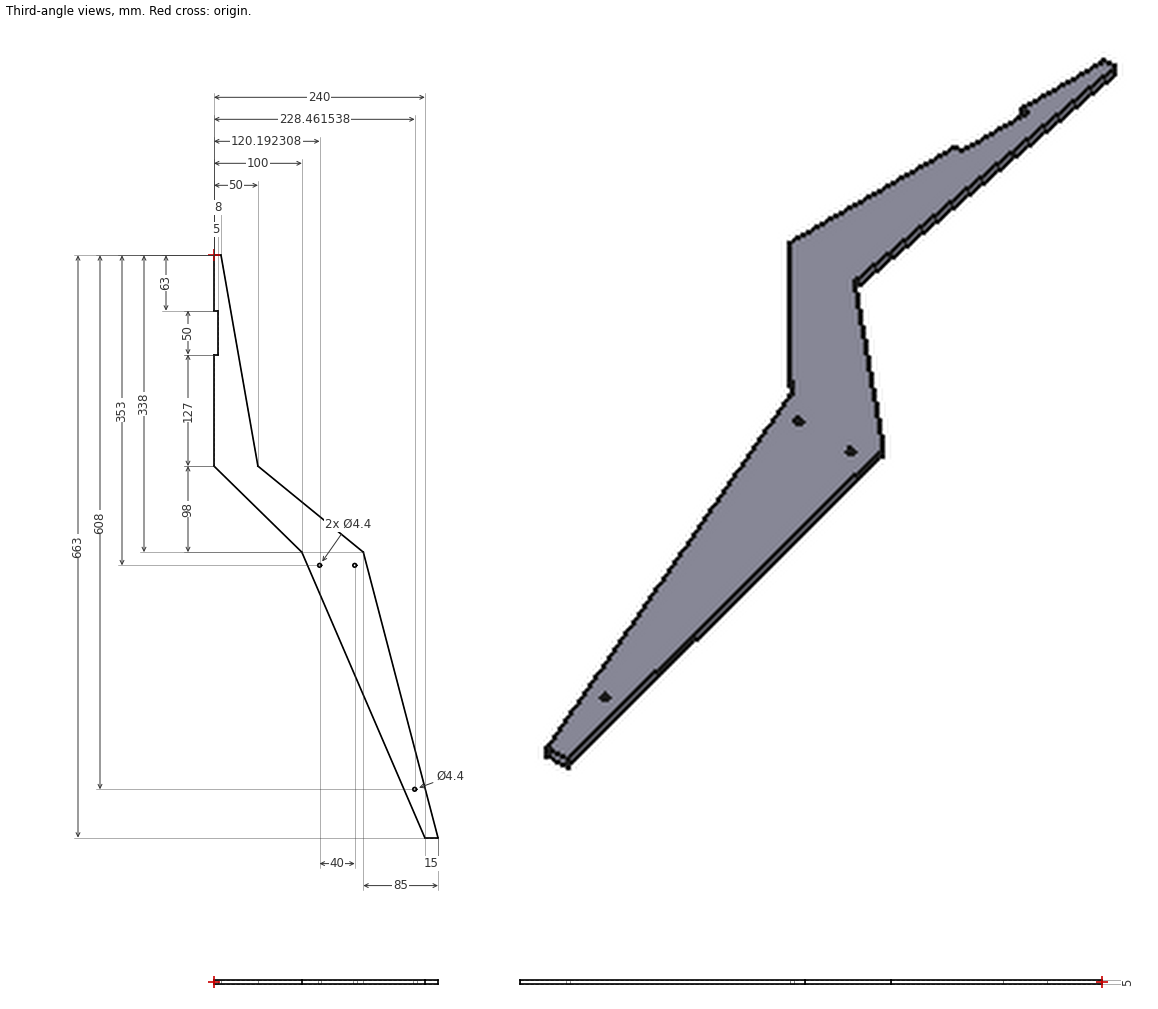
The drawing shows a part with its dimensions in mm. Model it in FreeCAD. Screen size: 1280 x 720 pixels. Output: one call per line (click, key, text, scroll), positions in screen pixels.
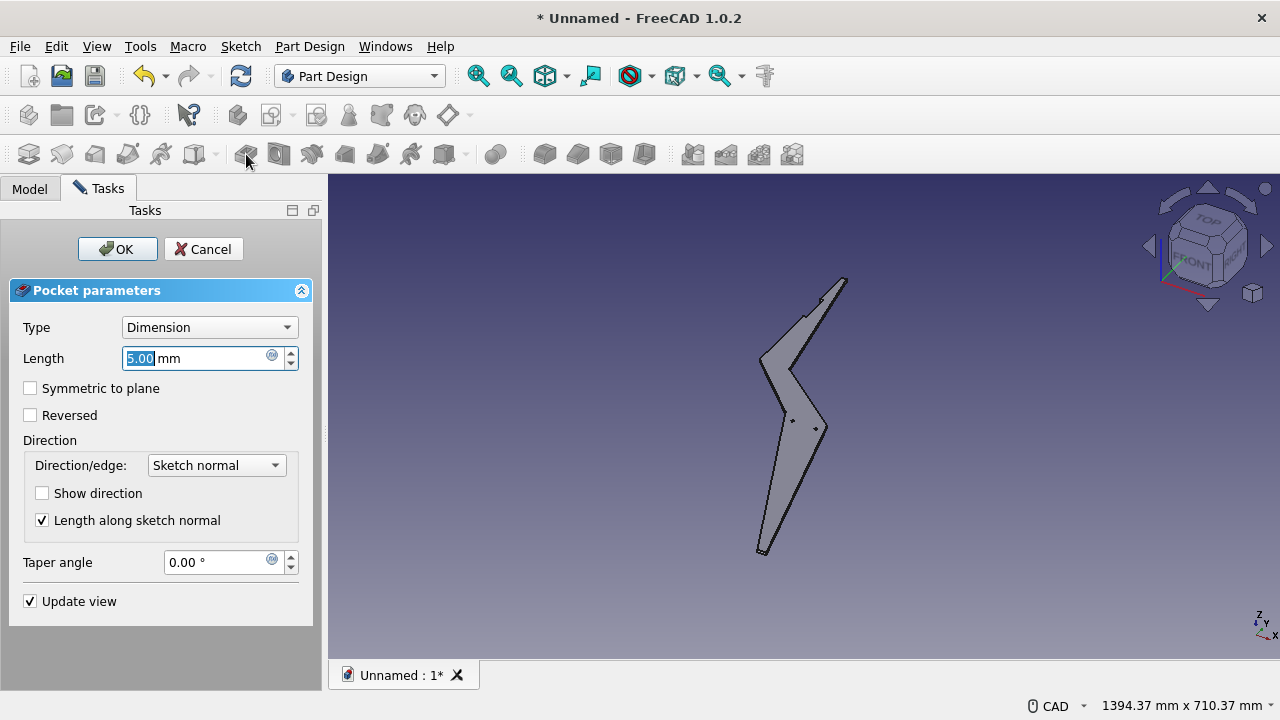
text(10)
key(Tab)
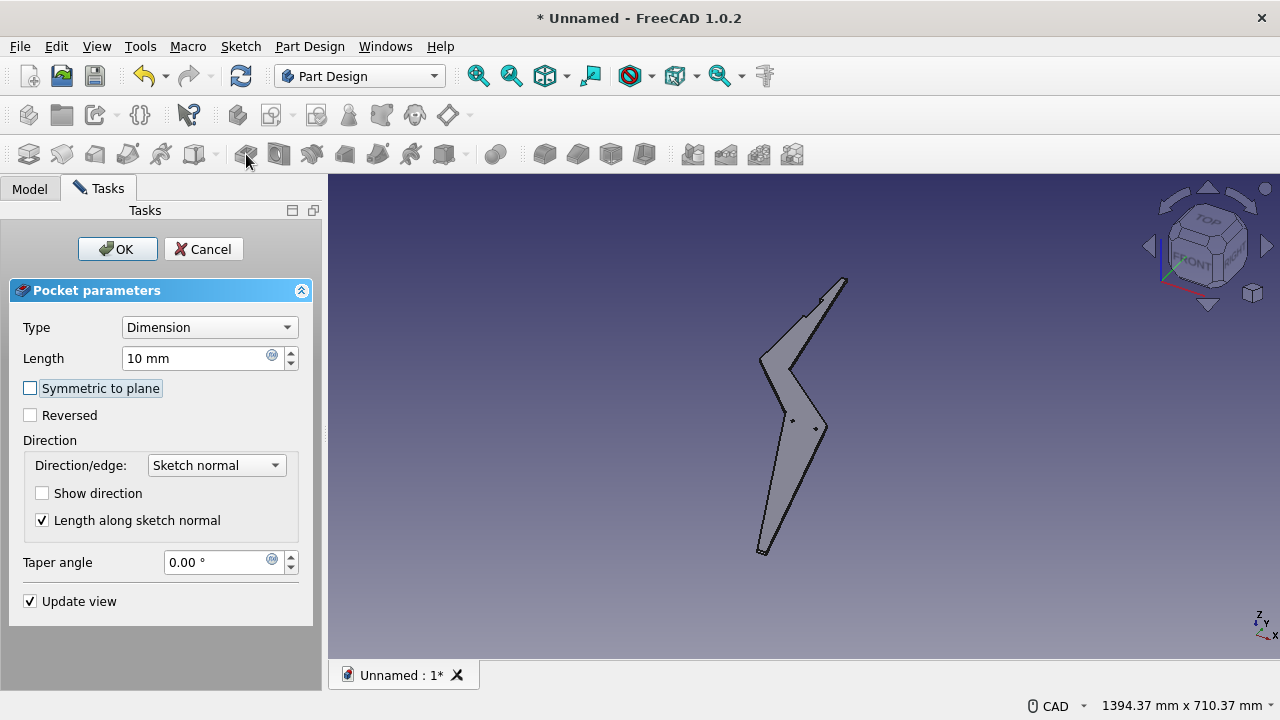
click(118, 249)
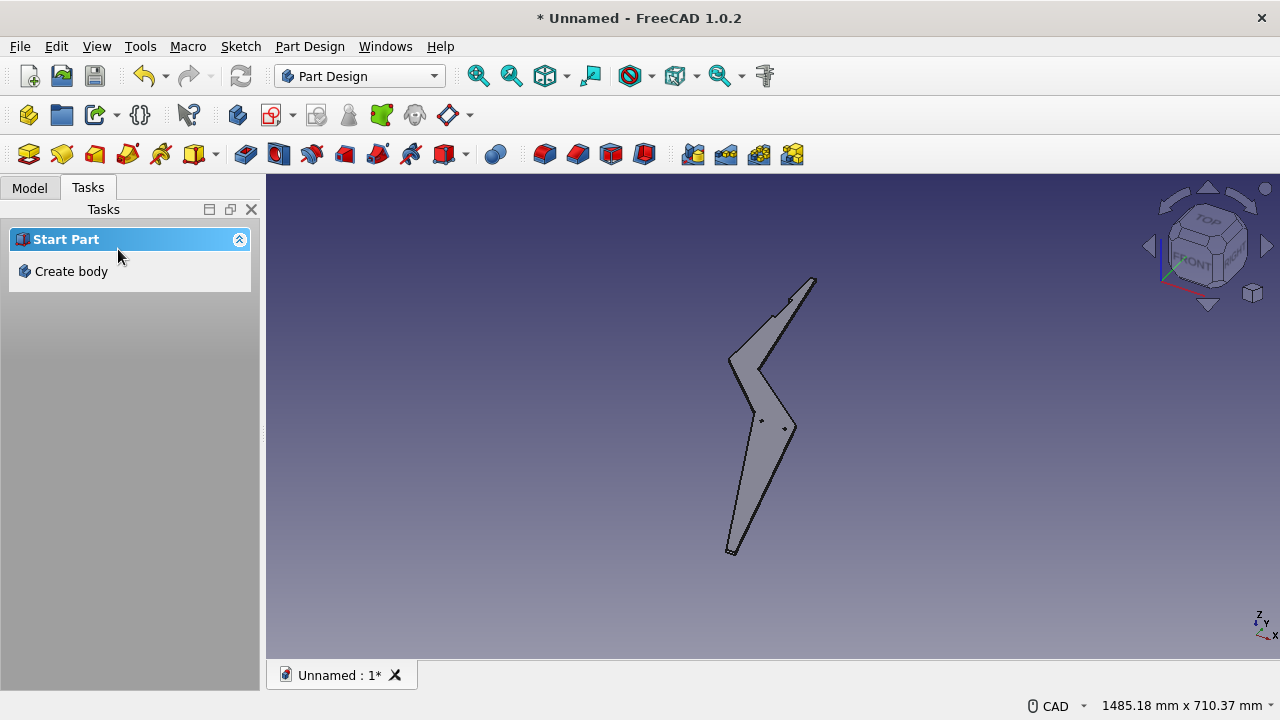
click(762, 453)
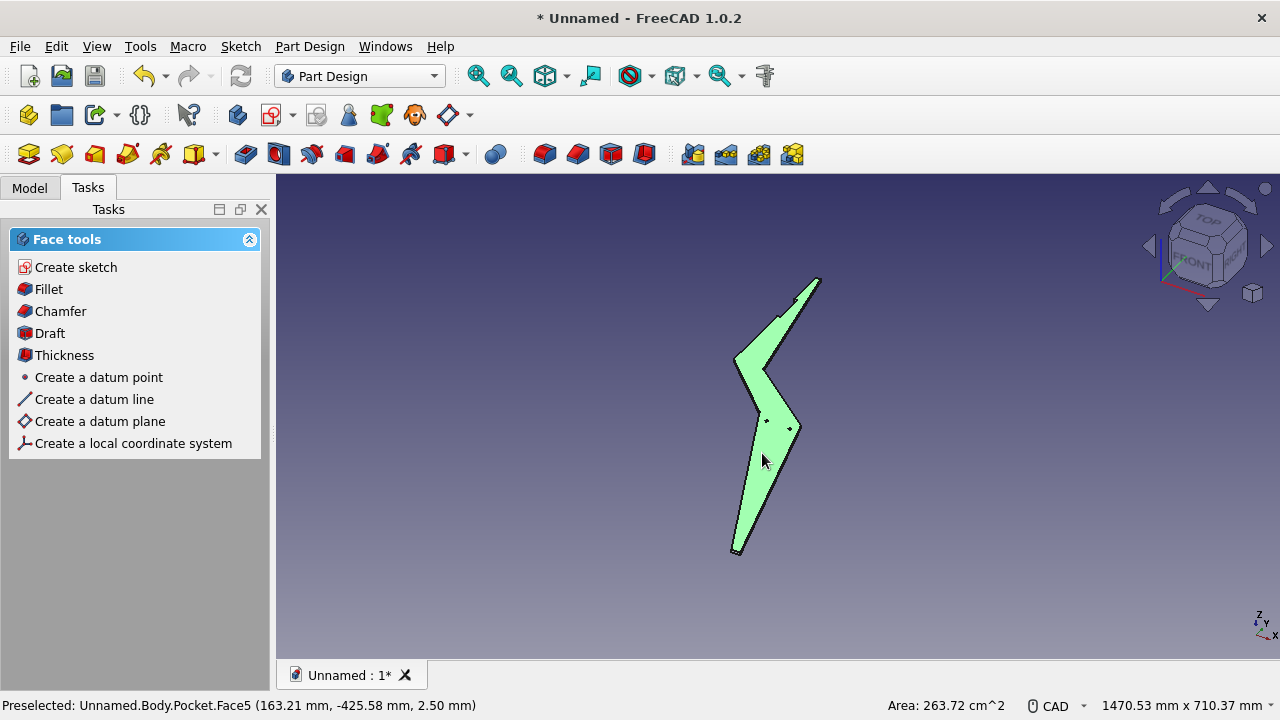
click(270, 116)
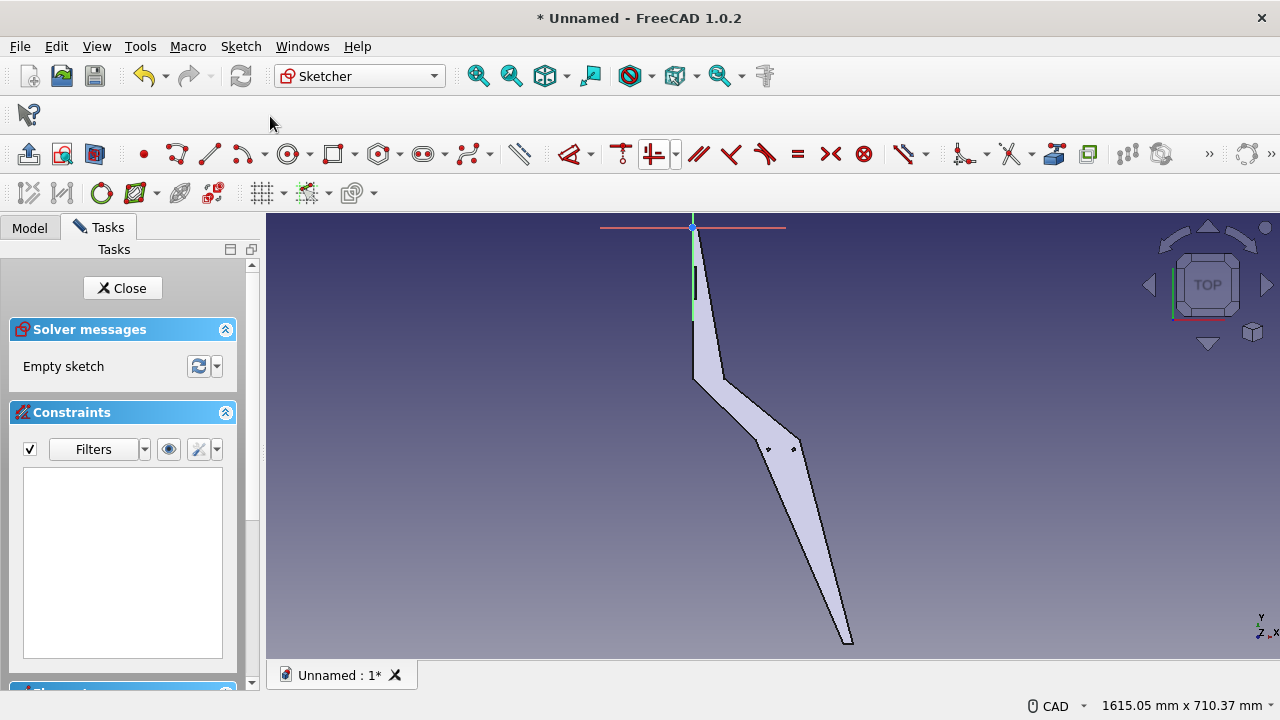
scroll(843, 619, up, 15)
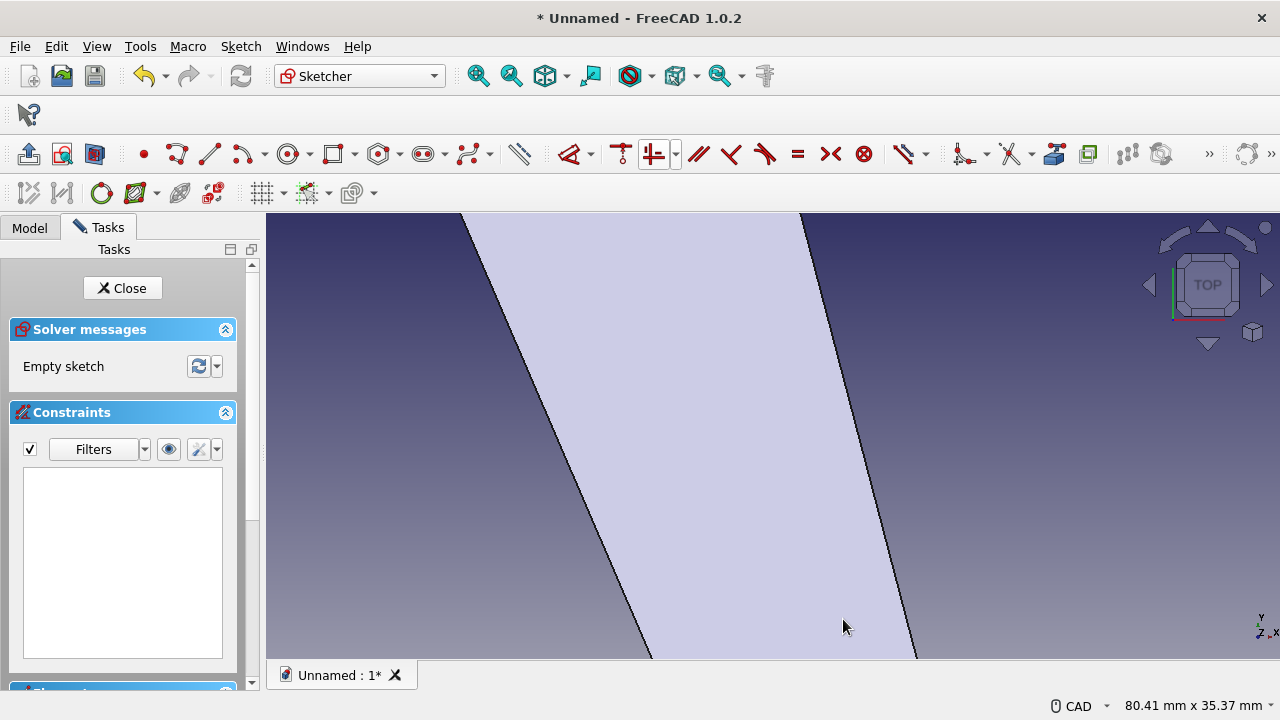
scroll(698, 407, up, 8)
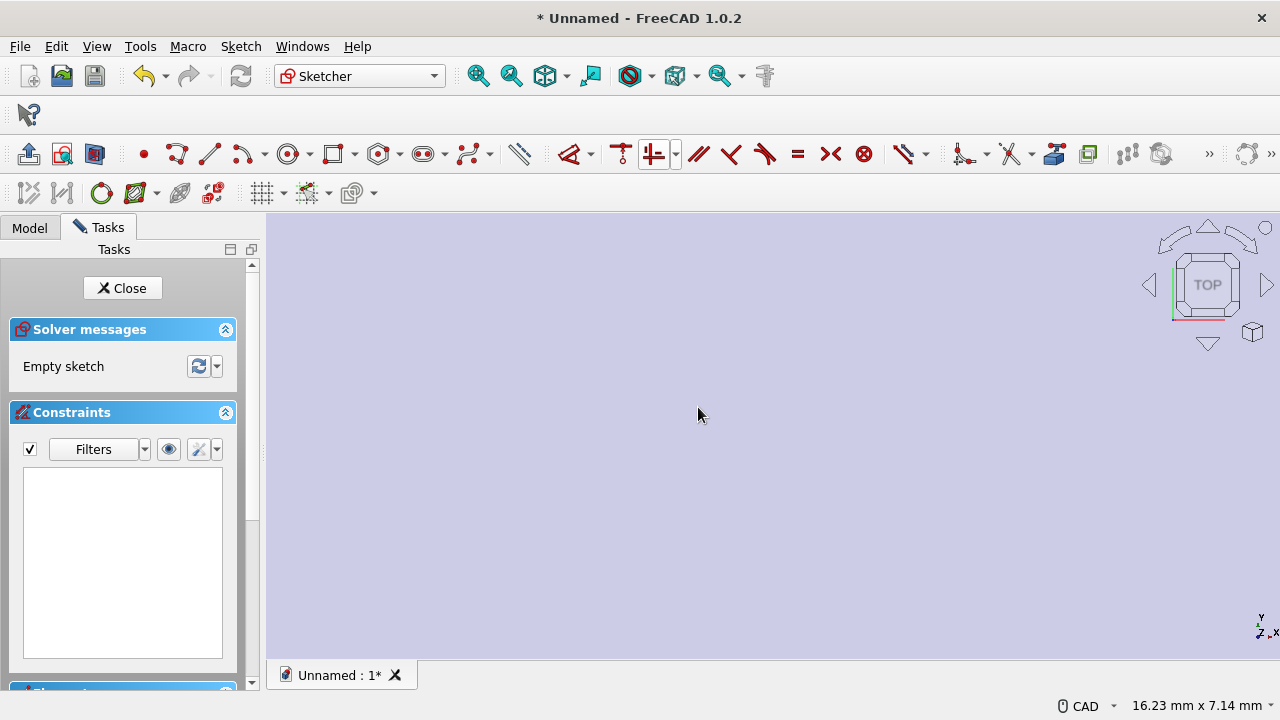
click(288, 154)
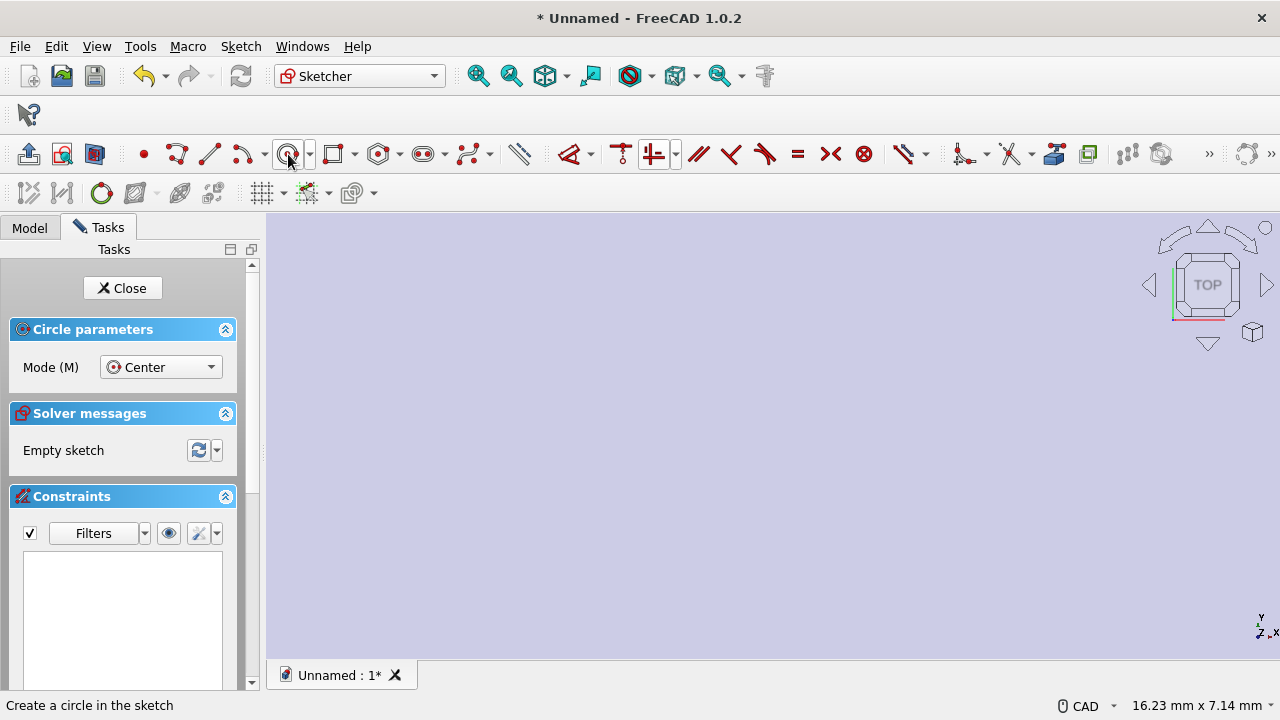
click(703, 434)
click(800, 337)
key(Escape)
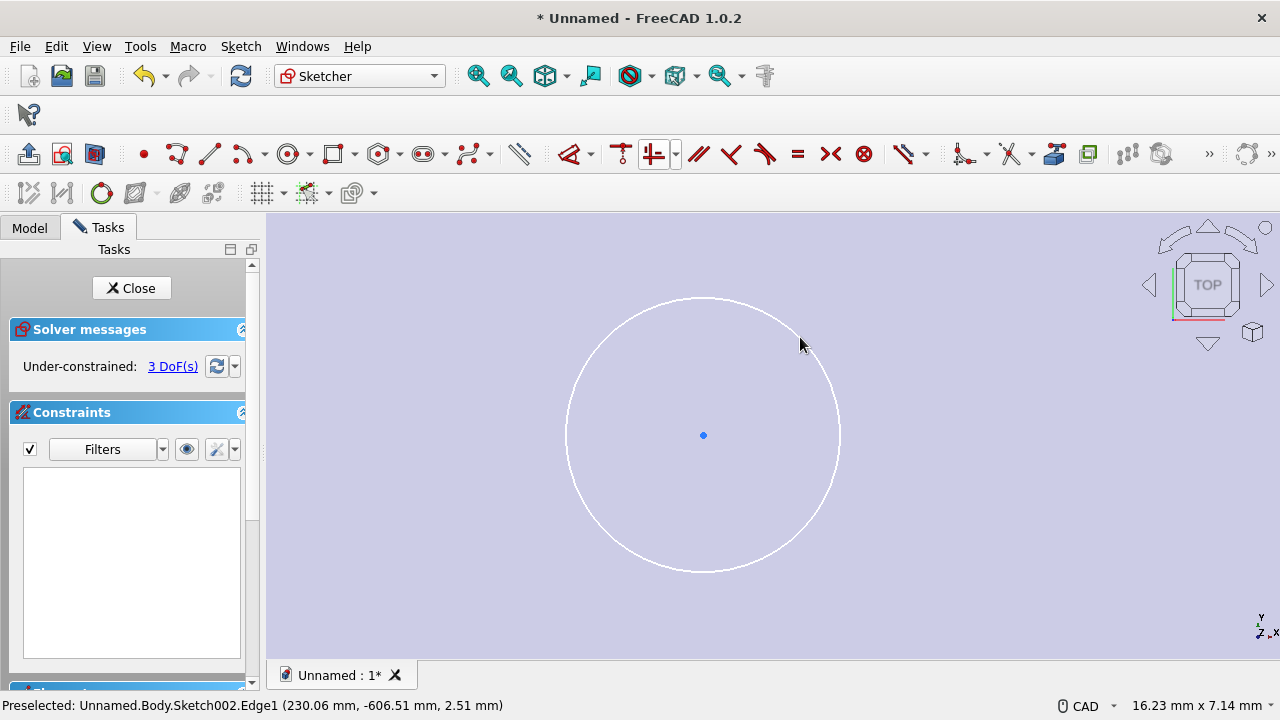
click(568, 154)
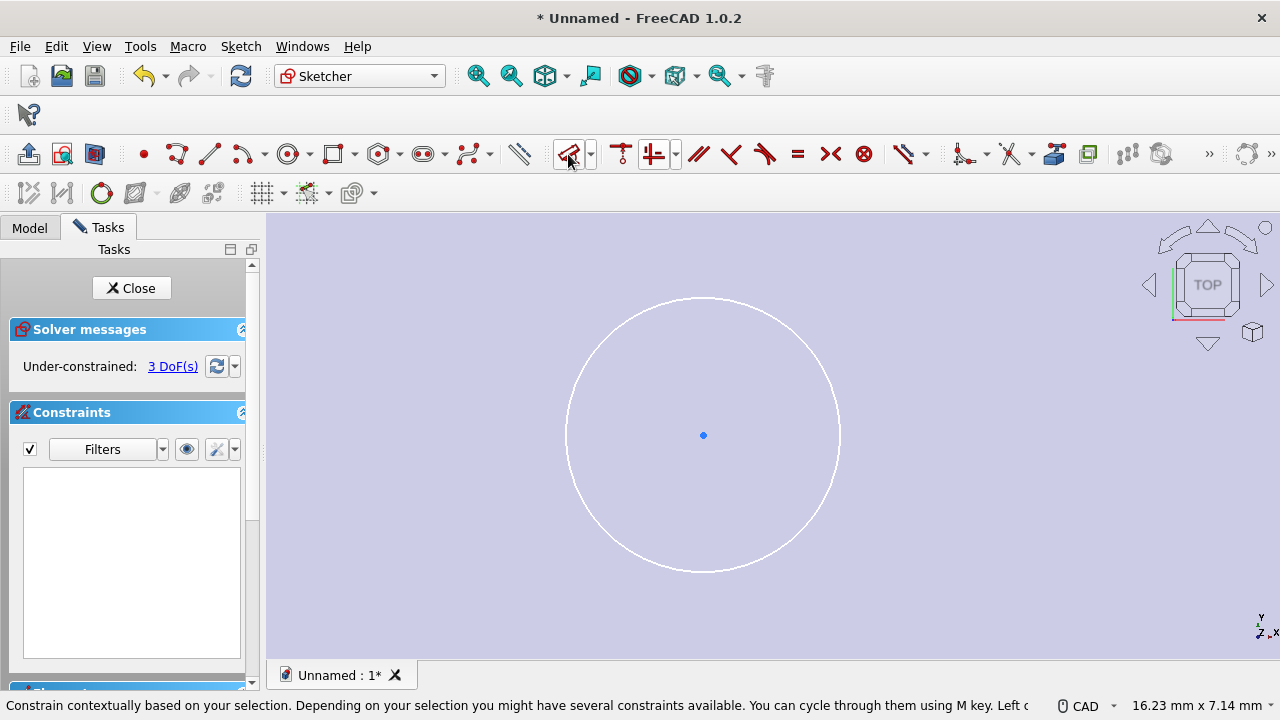
click(800, 338)
click(823, 315)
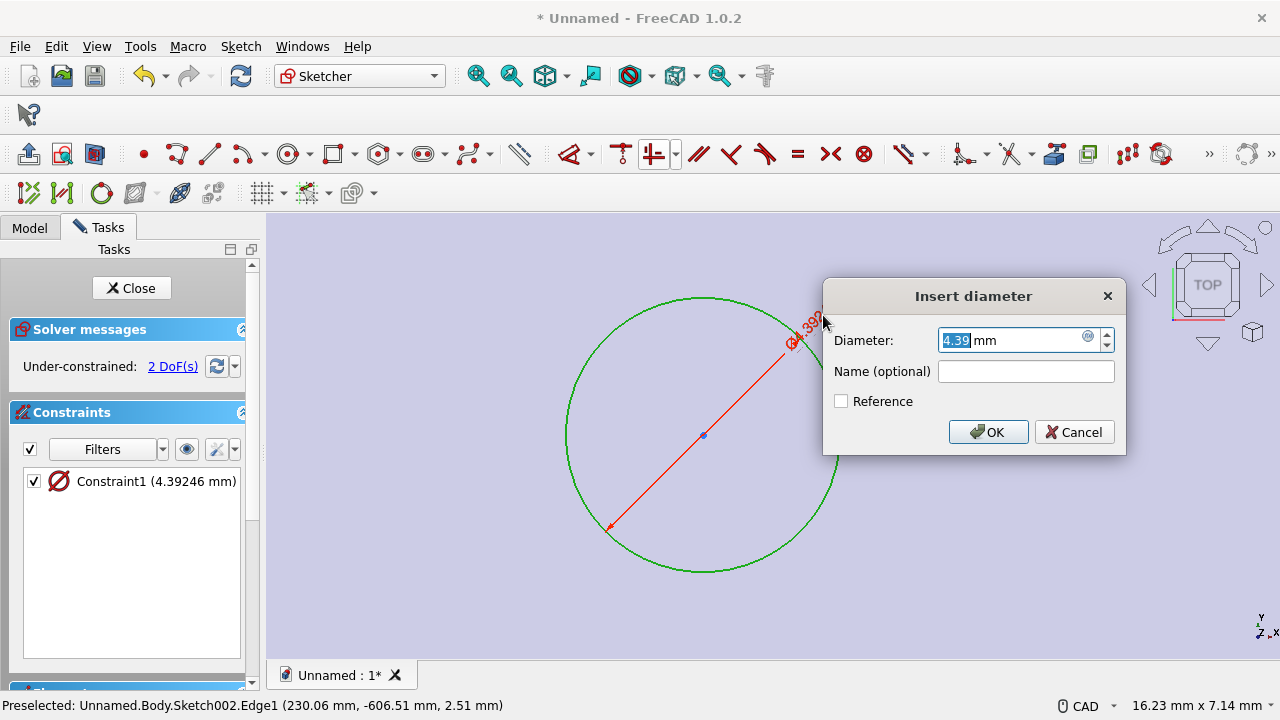
text(4.4)
key(Return)